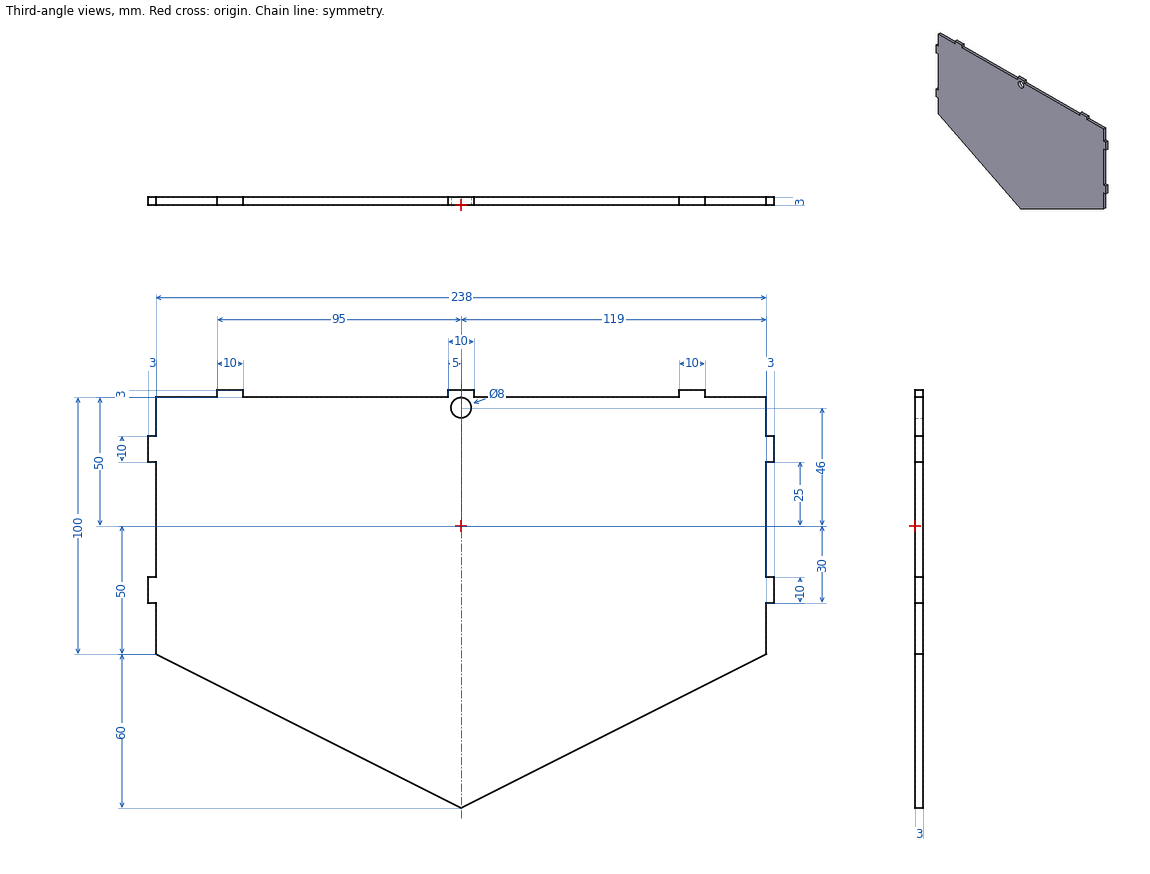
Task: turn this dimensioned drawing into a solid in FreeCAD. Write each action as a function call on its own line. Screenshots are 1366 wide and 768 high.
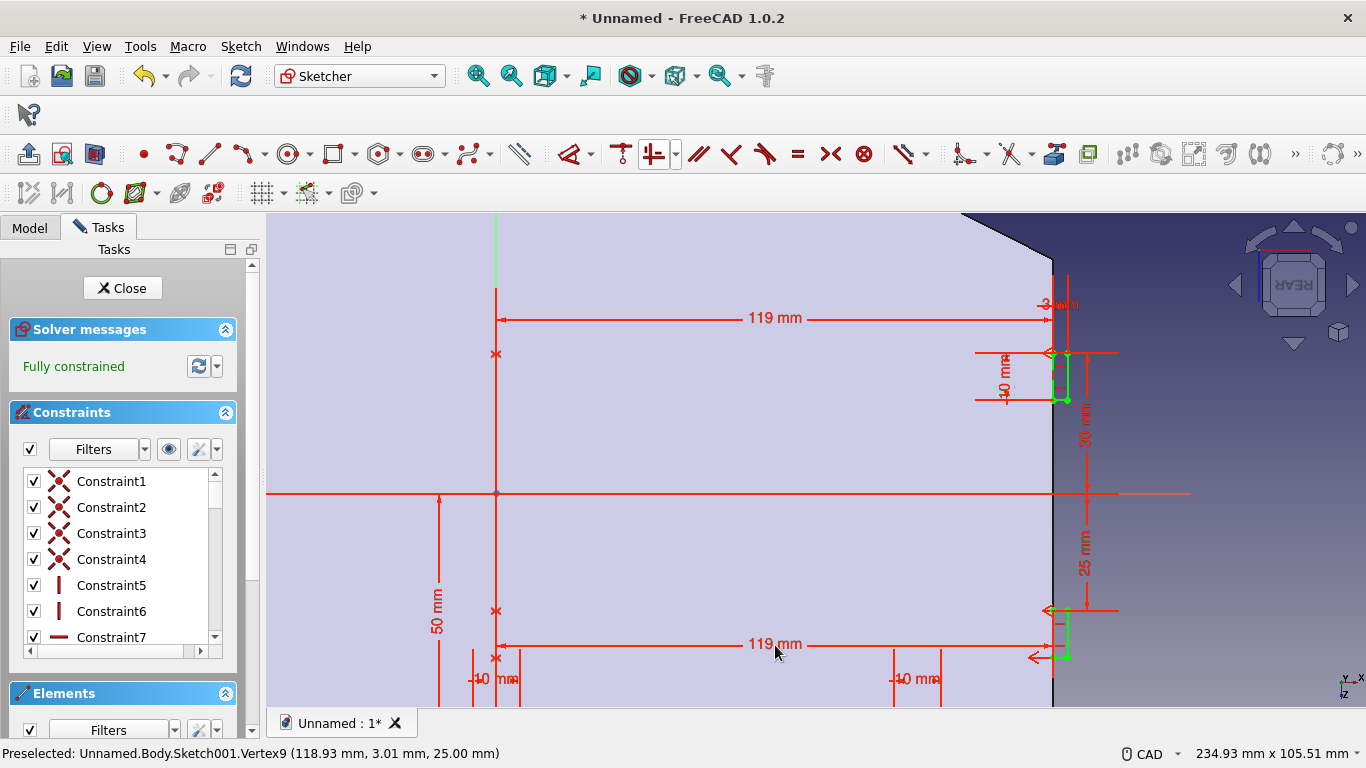
click(123, 288)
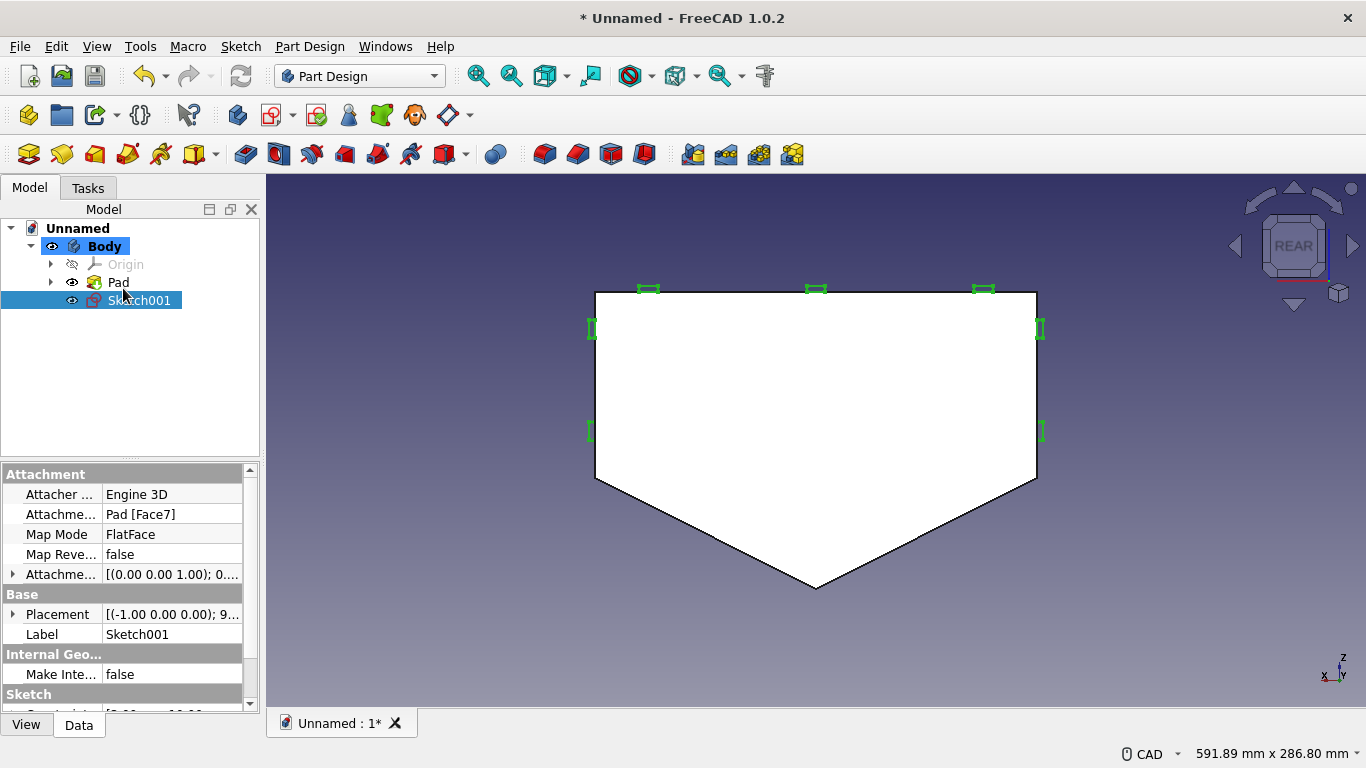
click(29, 154)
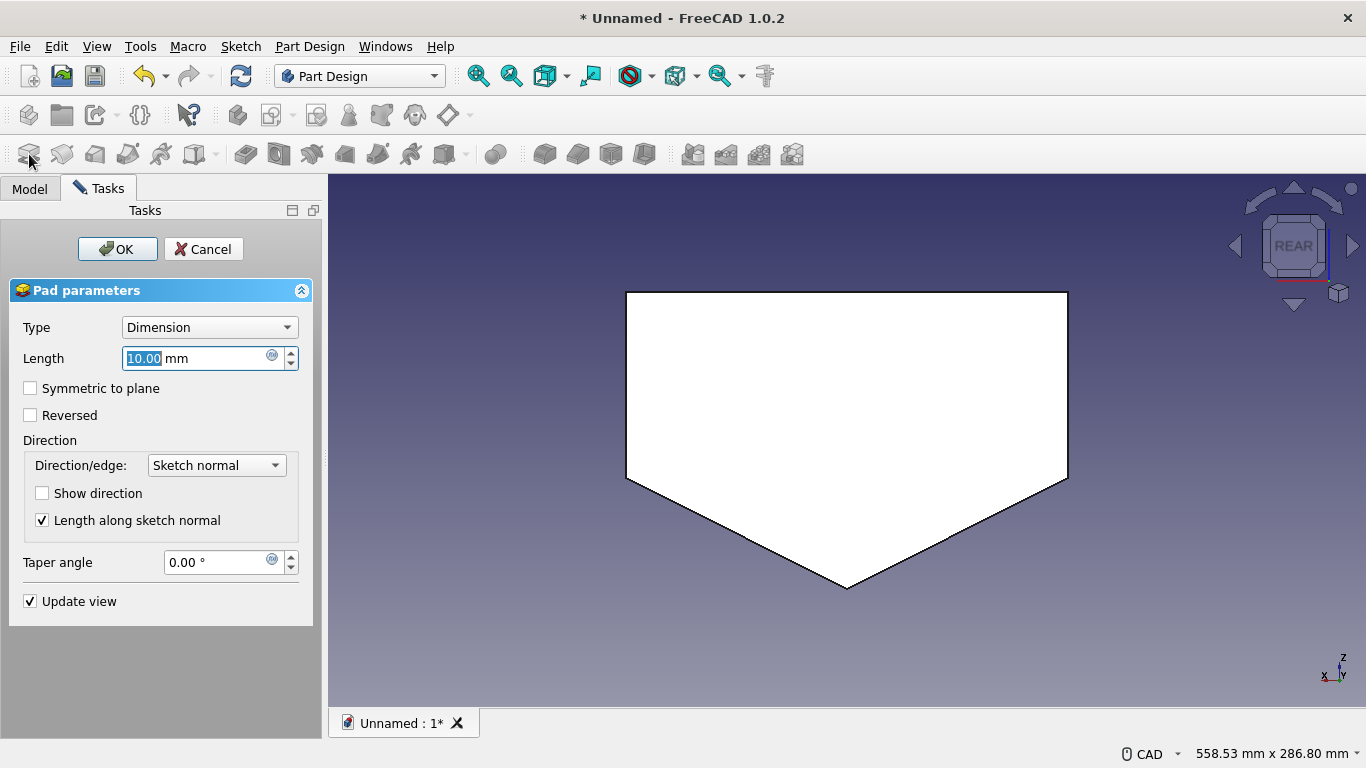
text(3)
key(Tab)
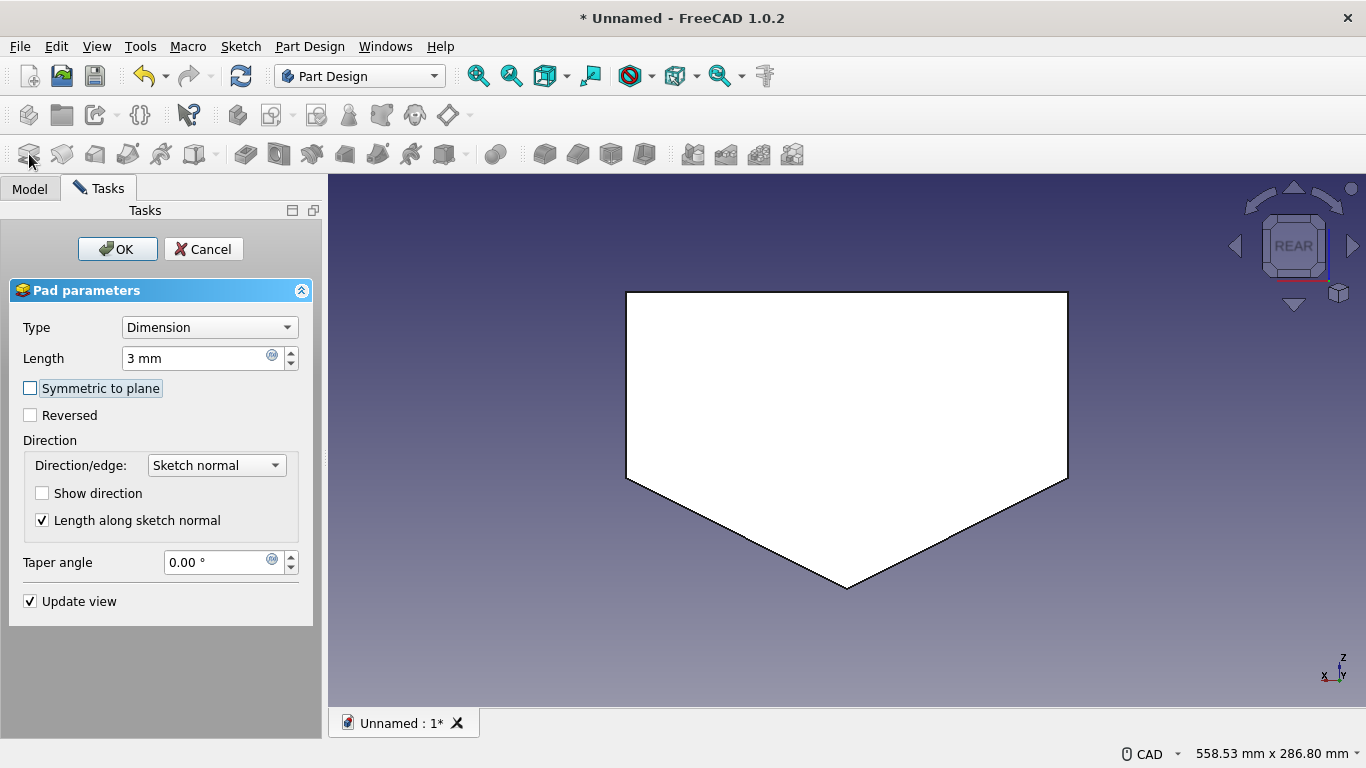
click(31, 415)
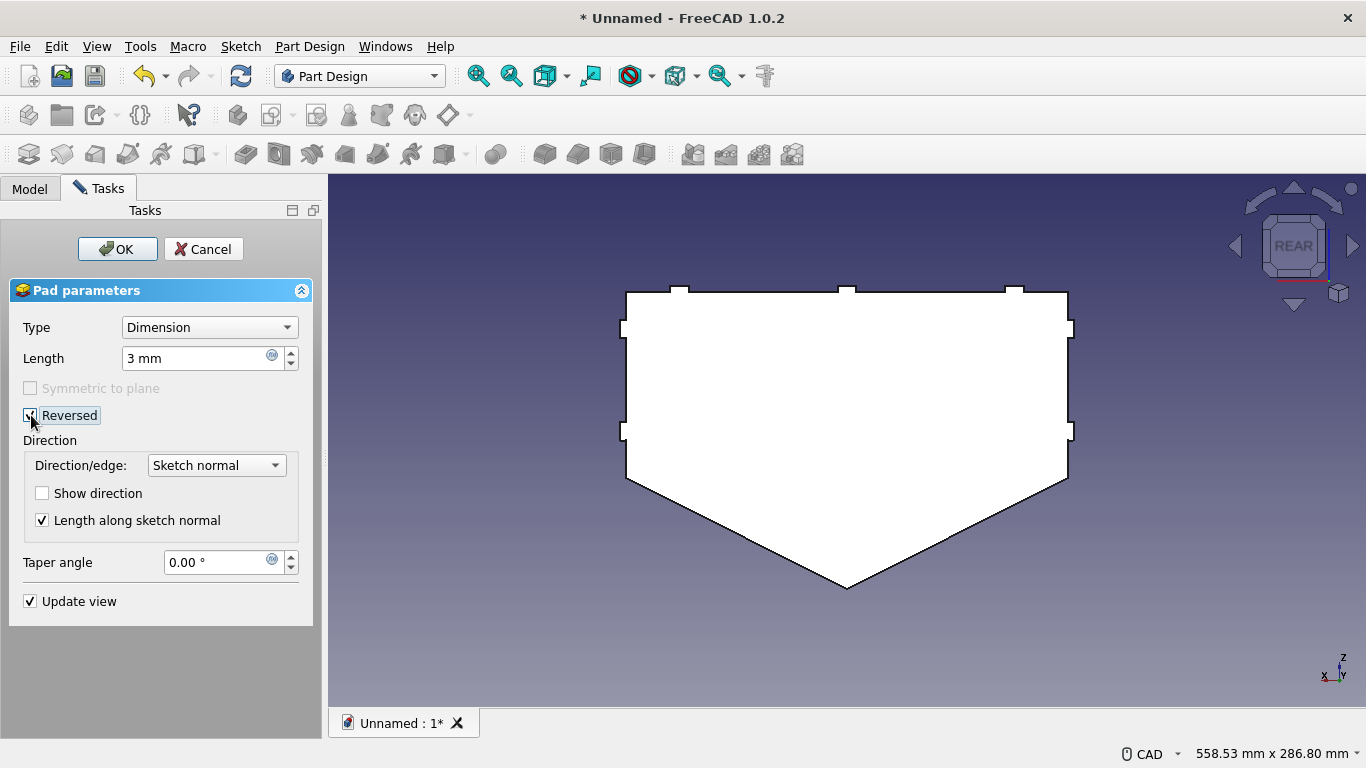
click(118, 249)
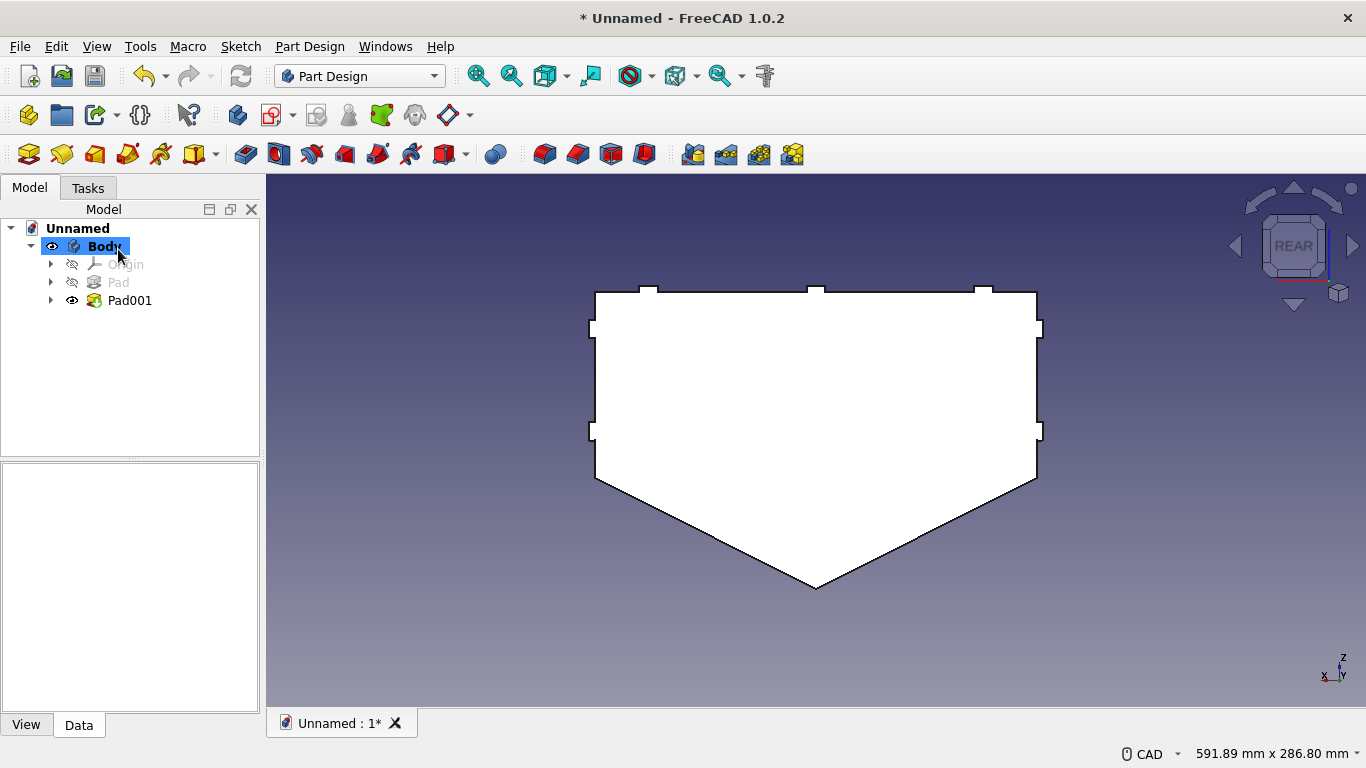
click(816, 437)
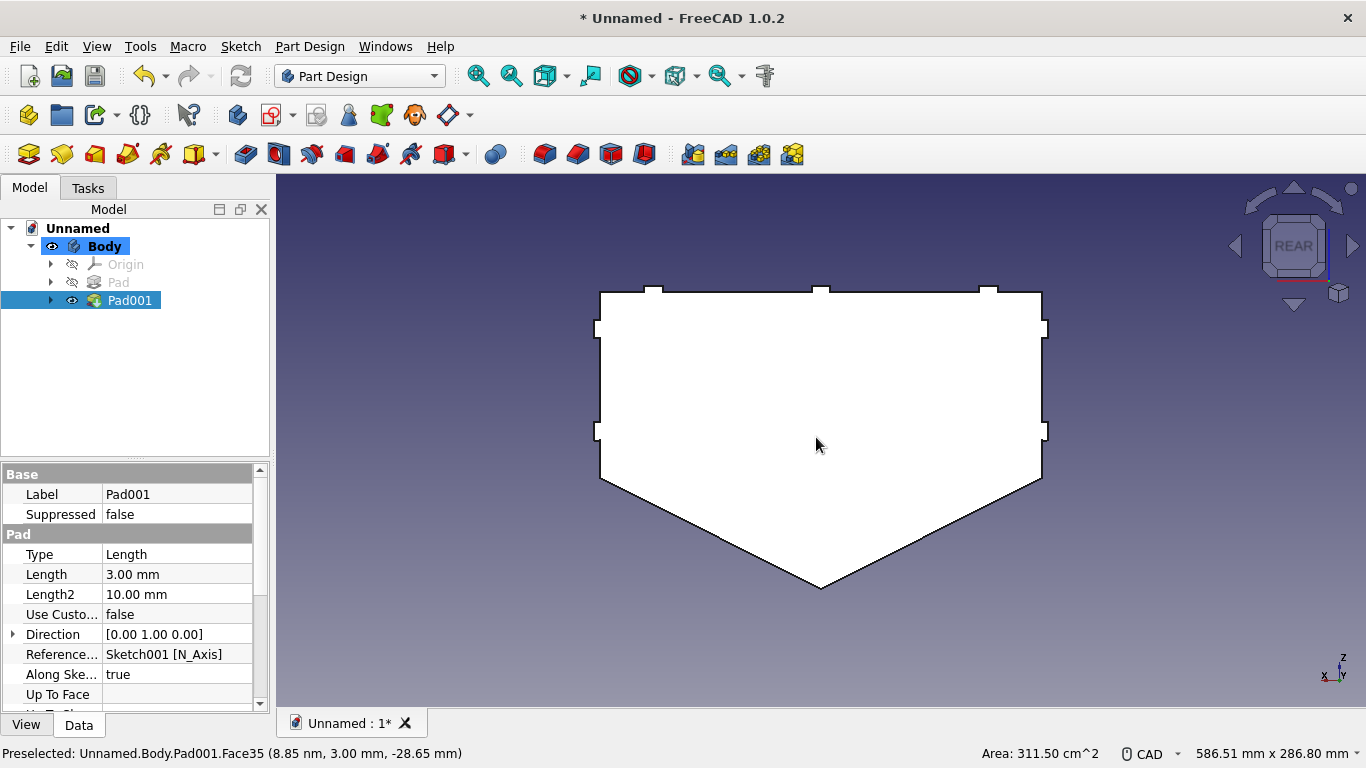
click(270, 116)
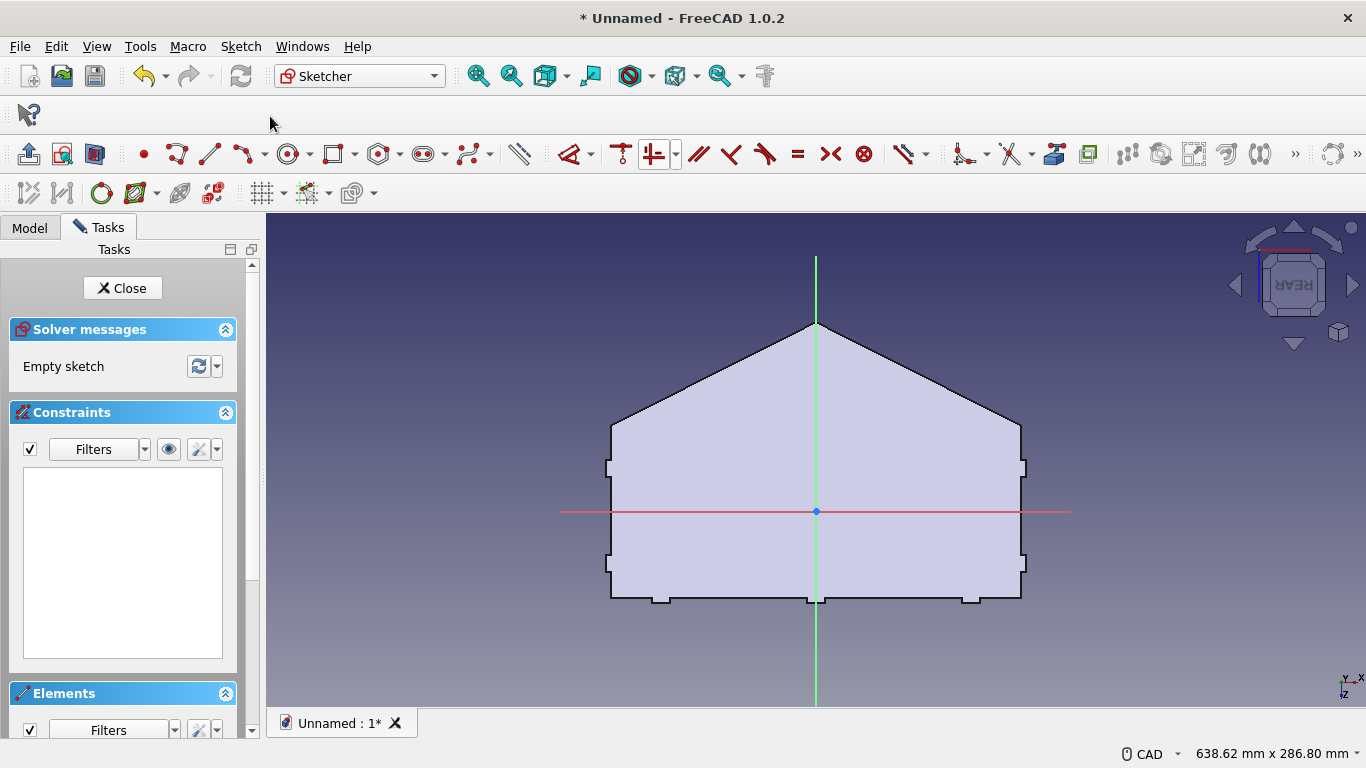
scroll(820, 598, up, 15)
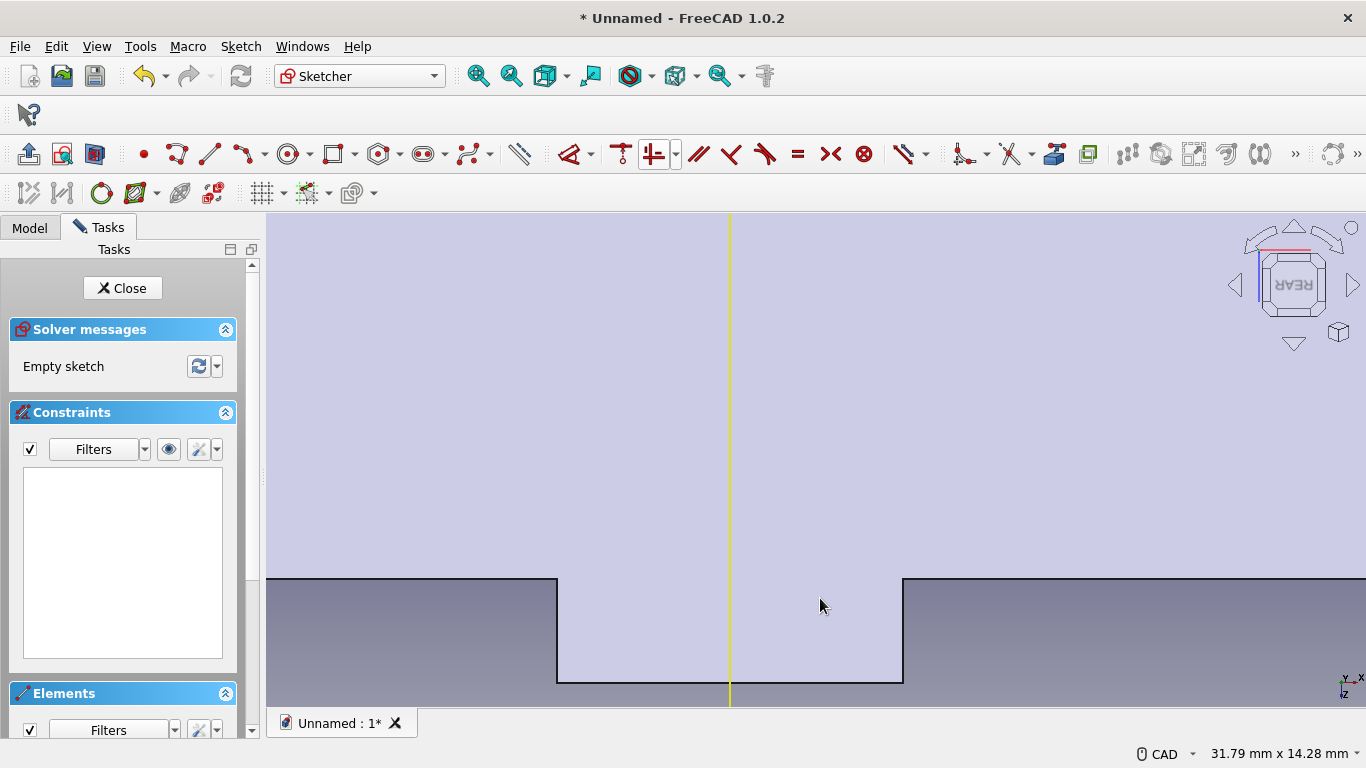
click(288, 154)